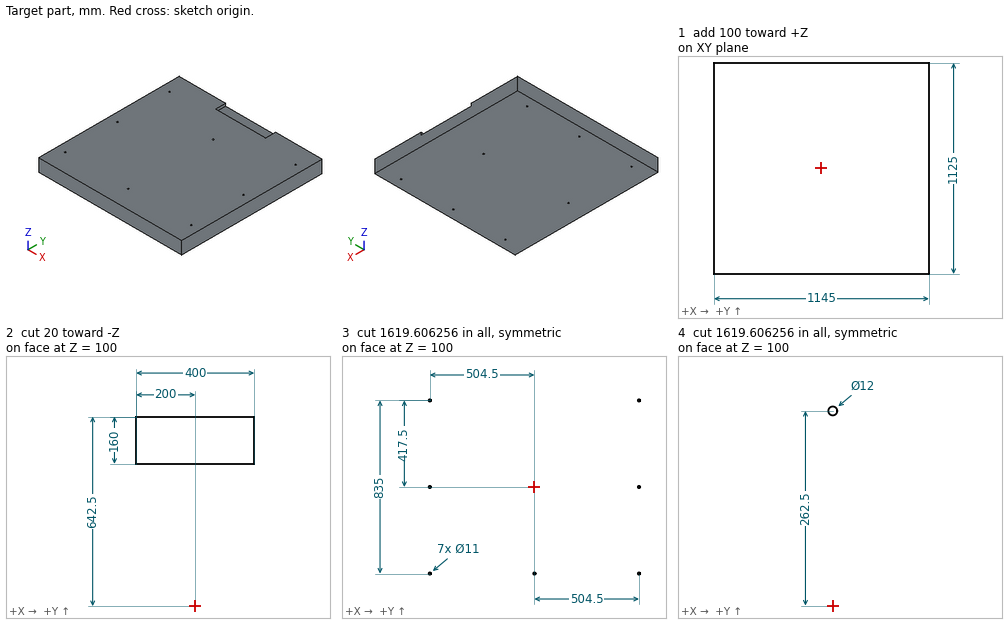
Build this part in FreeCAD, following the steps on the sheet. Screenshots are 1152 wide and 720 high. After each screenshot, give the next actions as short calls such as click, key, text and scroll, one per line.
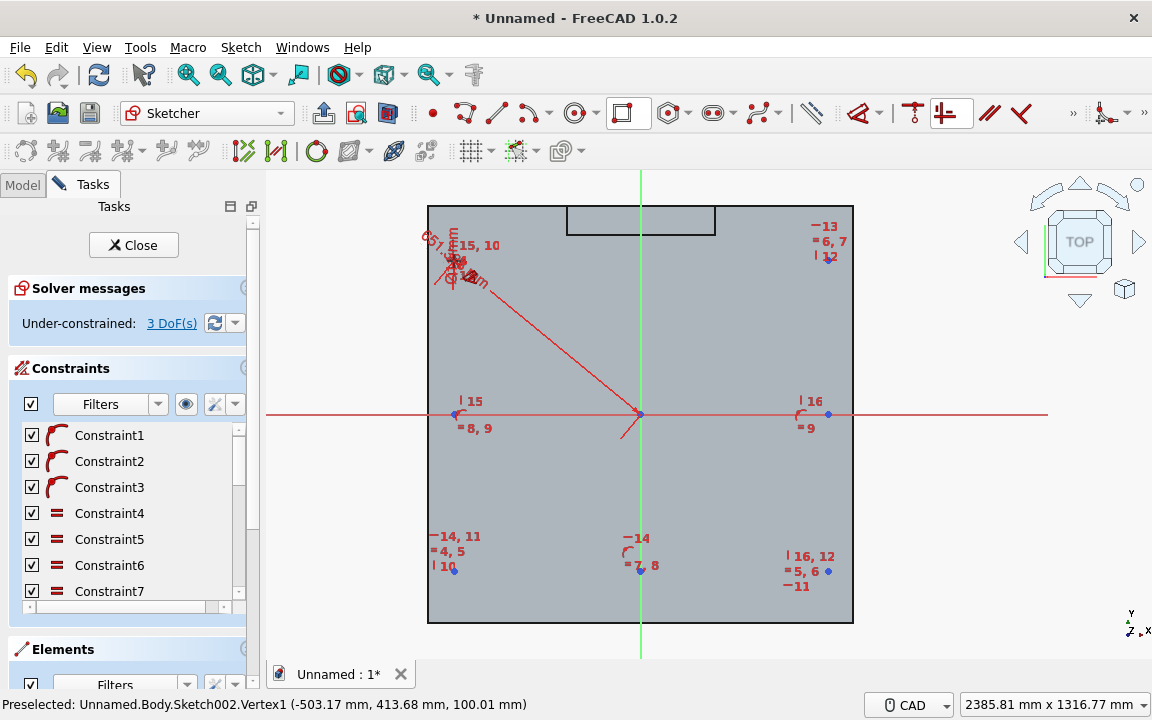
click(454, 571)
click(420, 345)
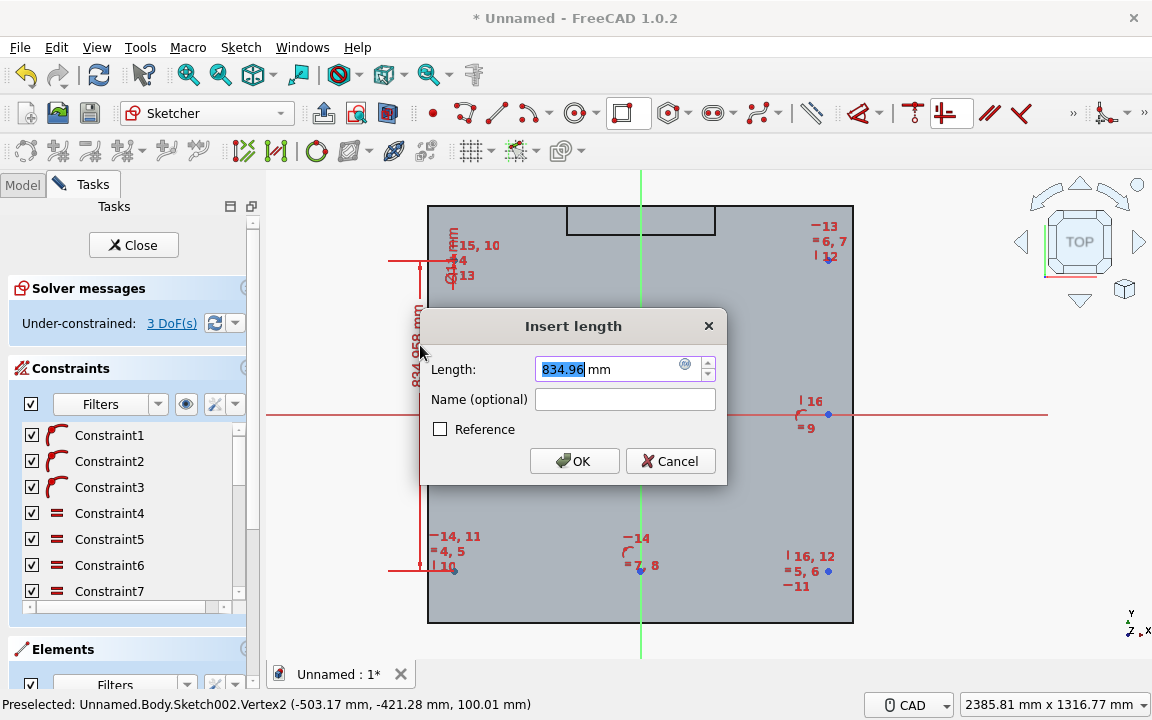
text(835)
key(Return)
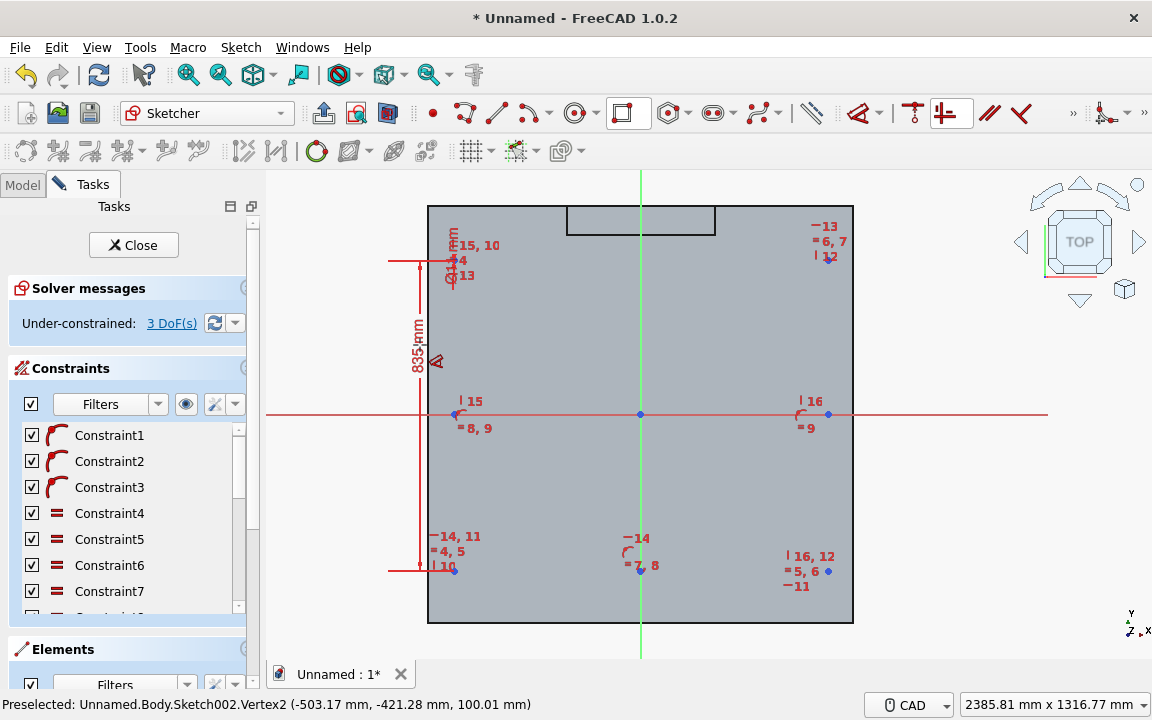
click(454, 261)
click(547, 227)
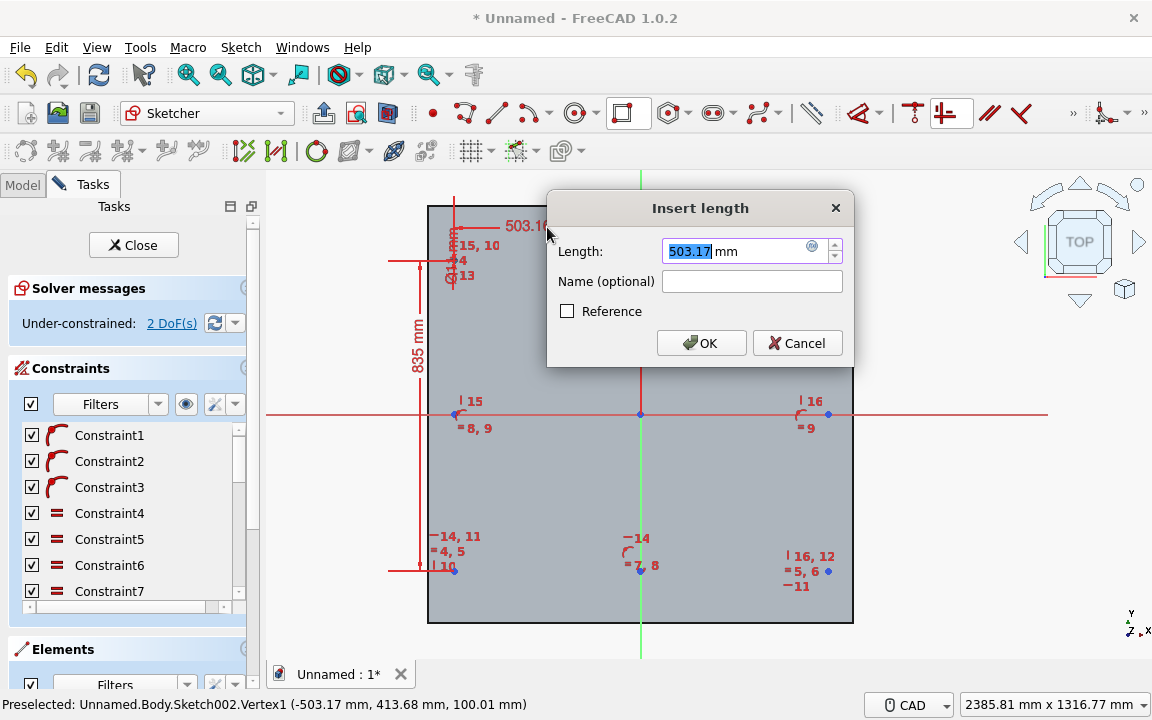
text(504.5)
key(Return)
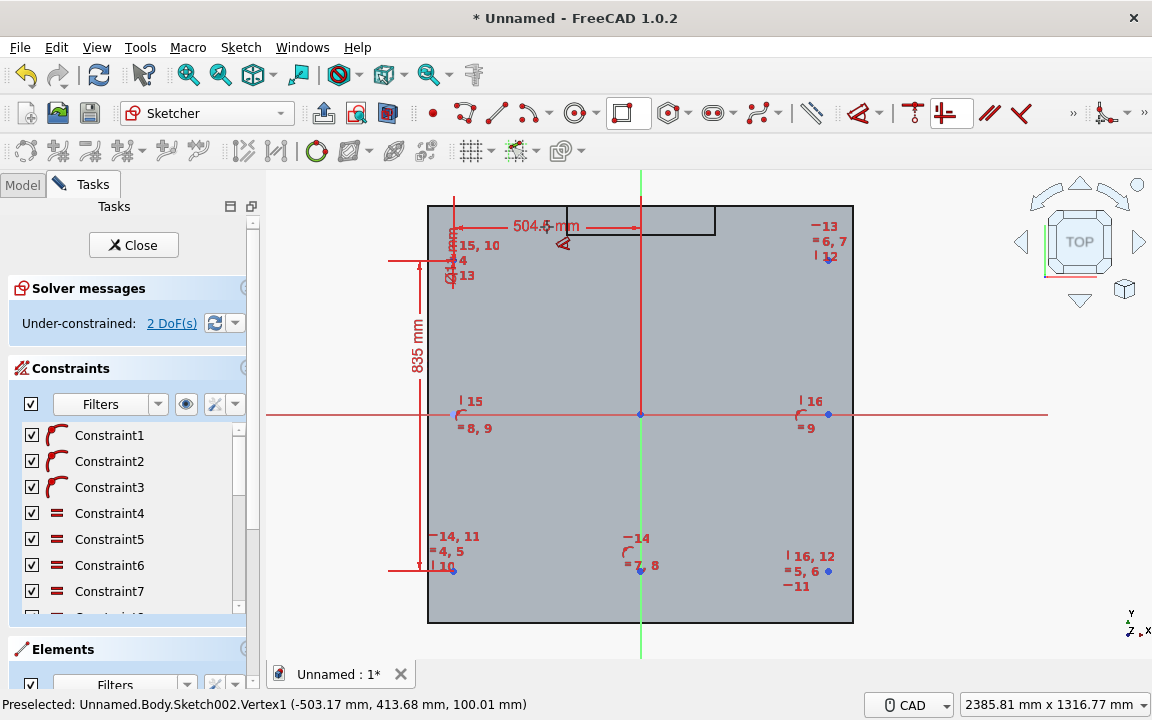
click(454, 261)
click(420, 302)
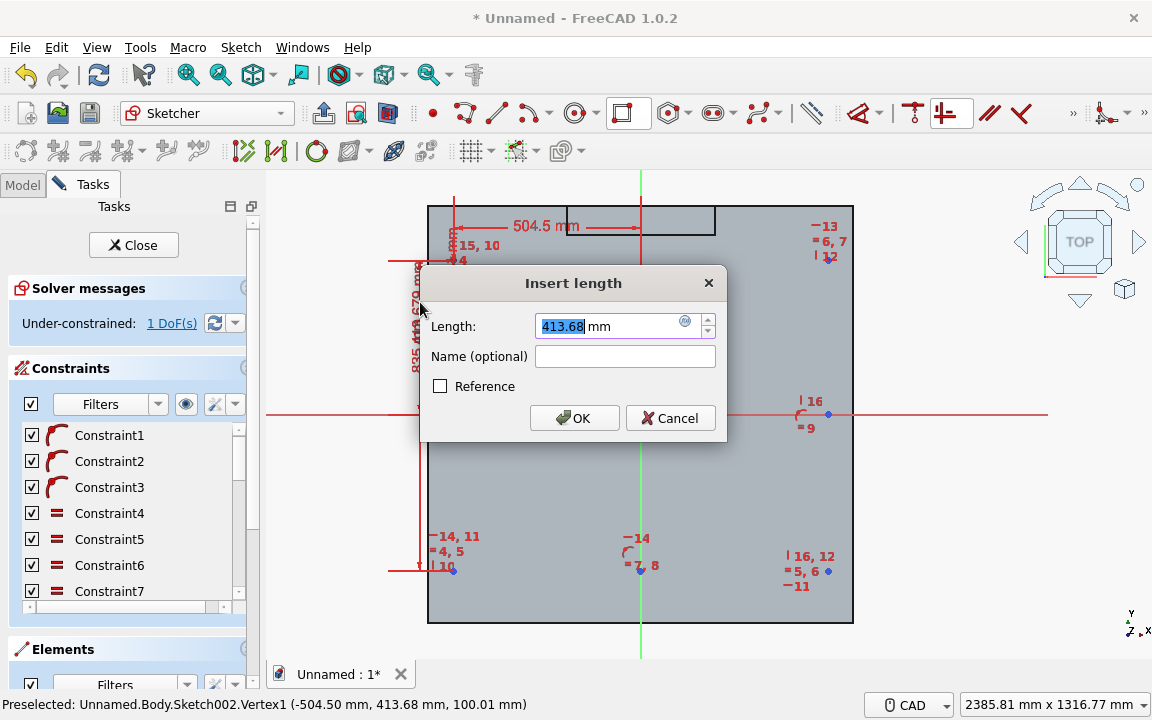
text(417.5)
key(Return)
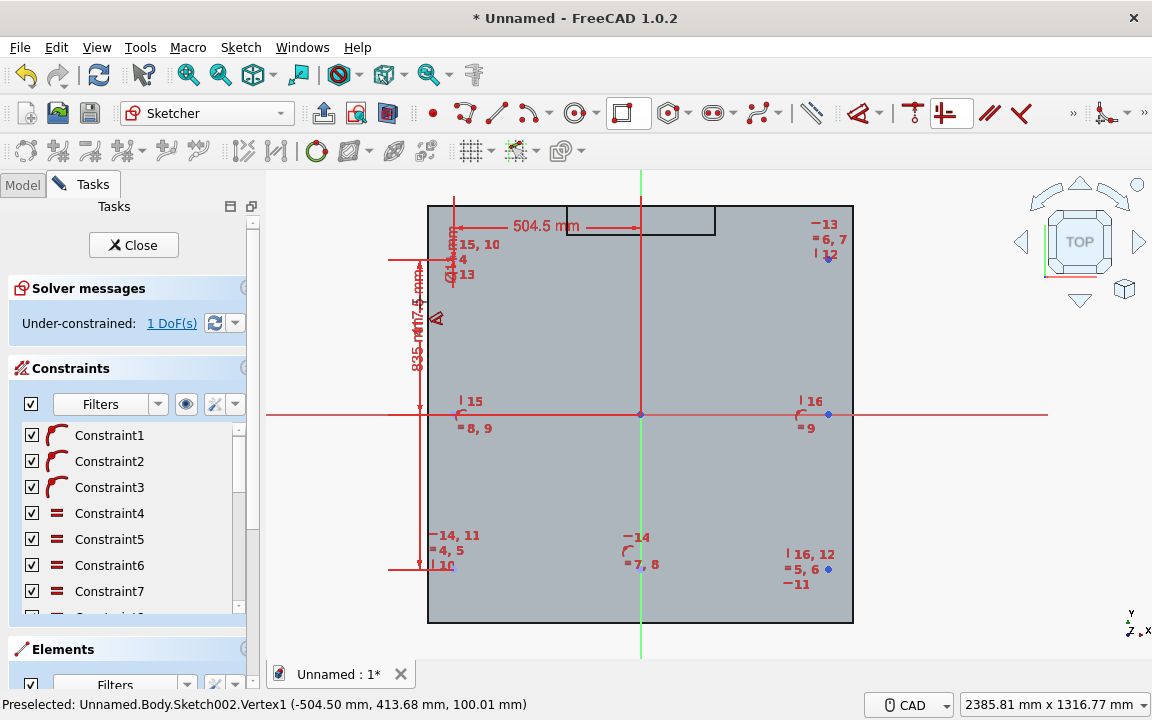
click(828, 570)
click(734, 604)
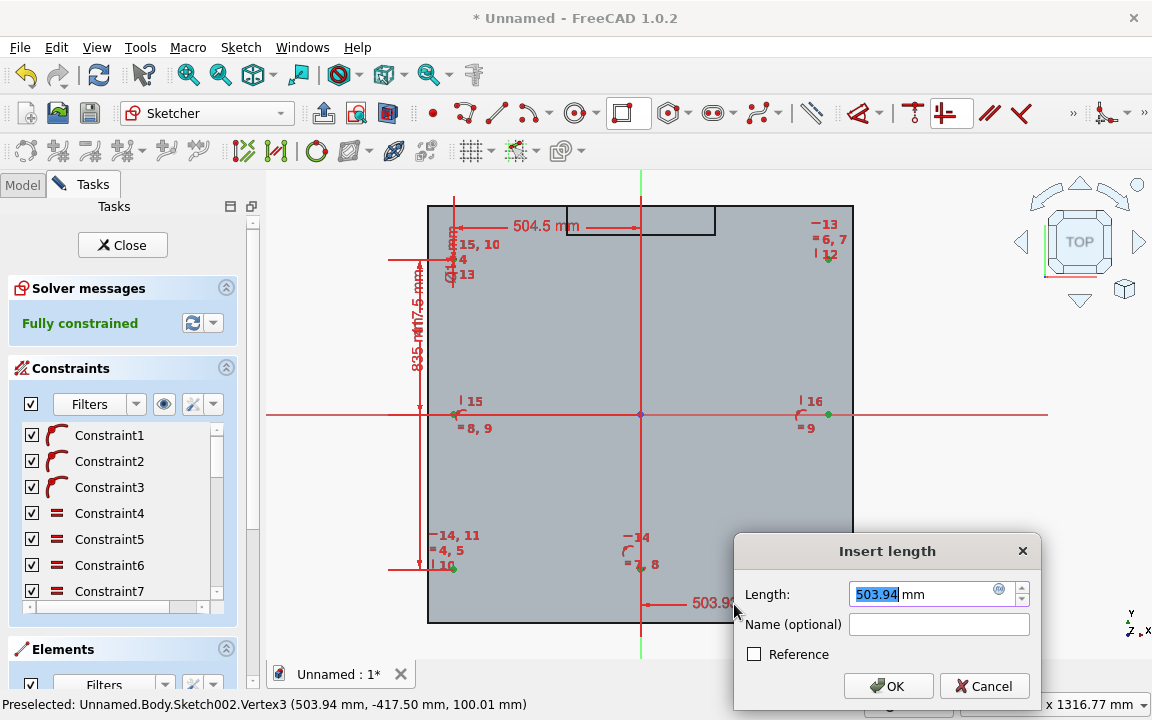
text(504.5)
key(Return)
key(Escape)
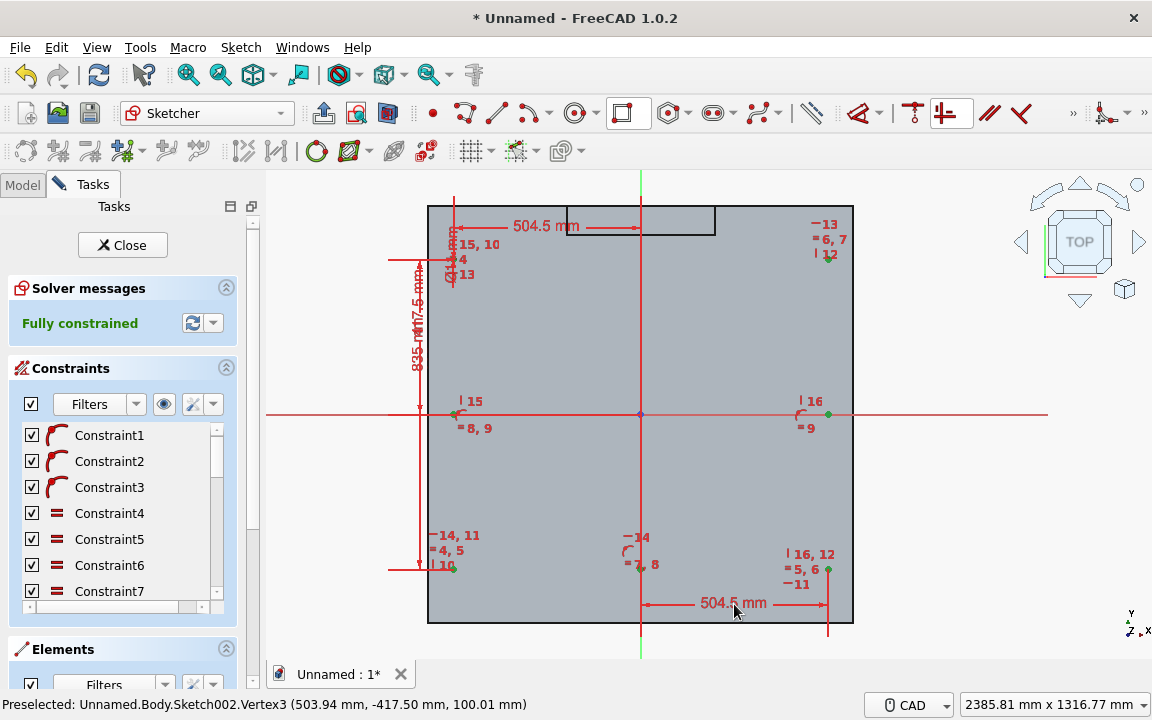
click(123, 245)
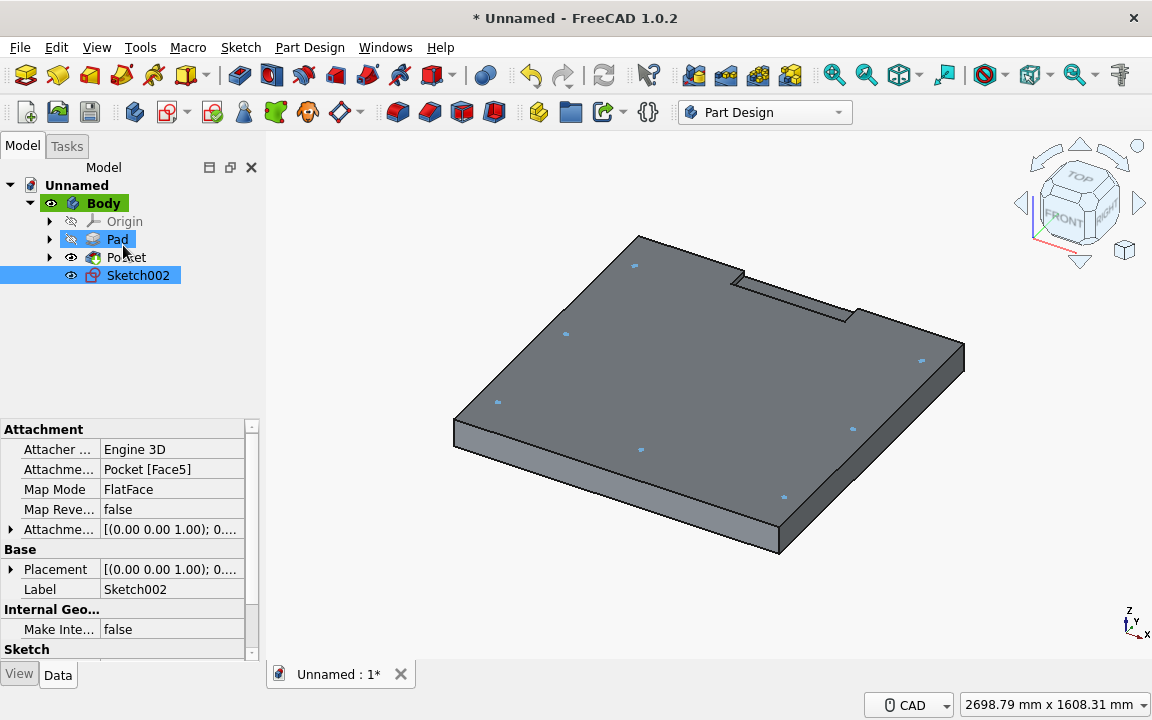
click(240, 76)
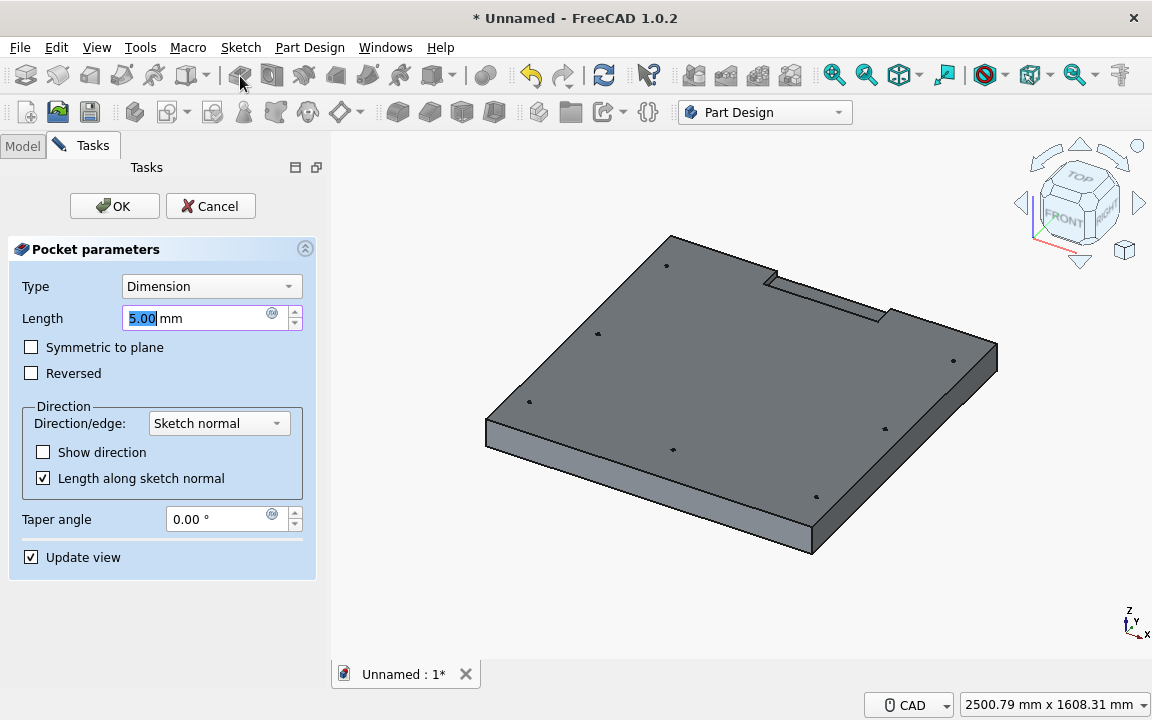
text(1619.606256)
key(Tab)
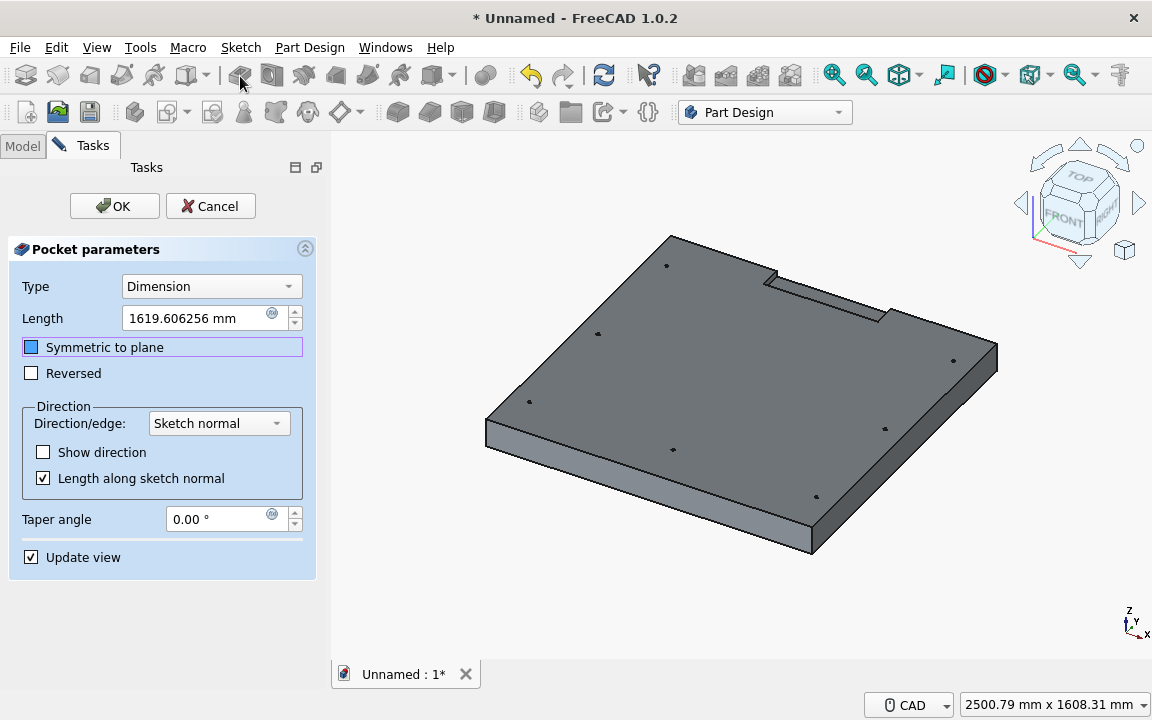
click(30, 347)